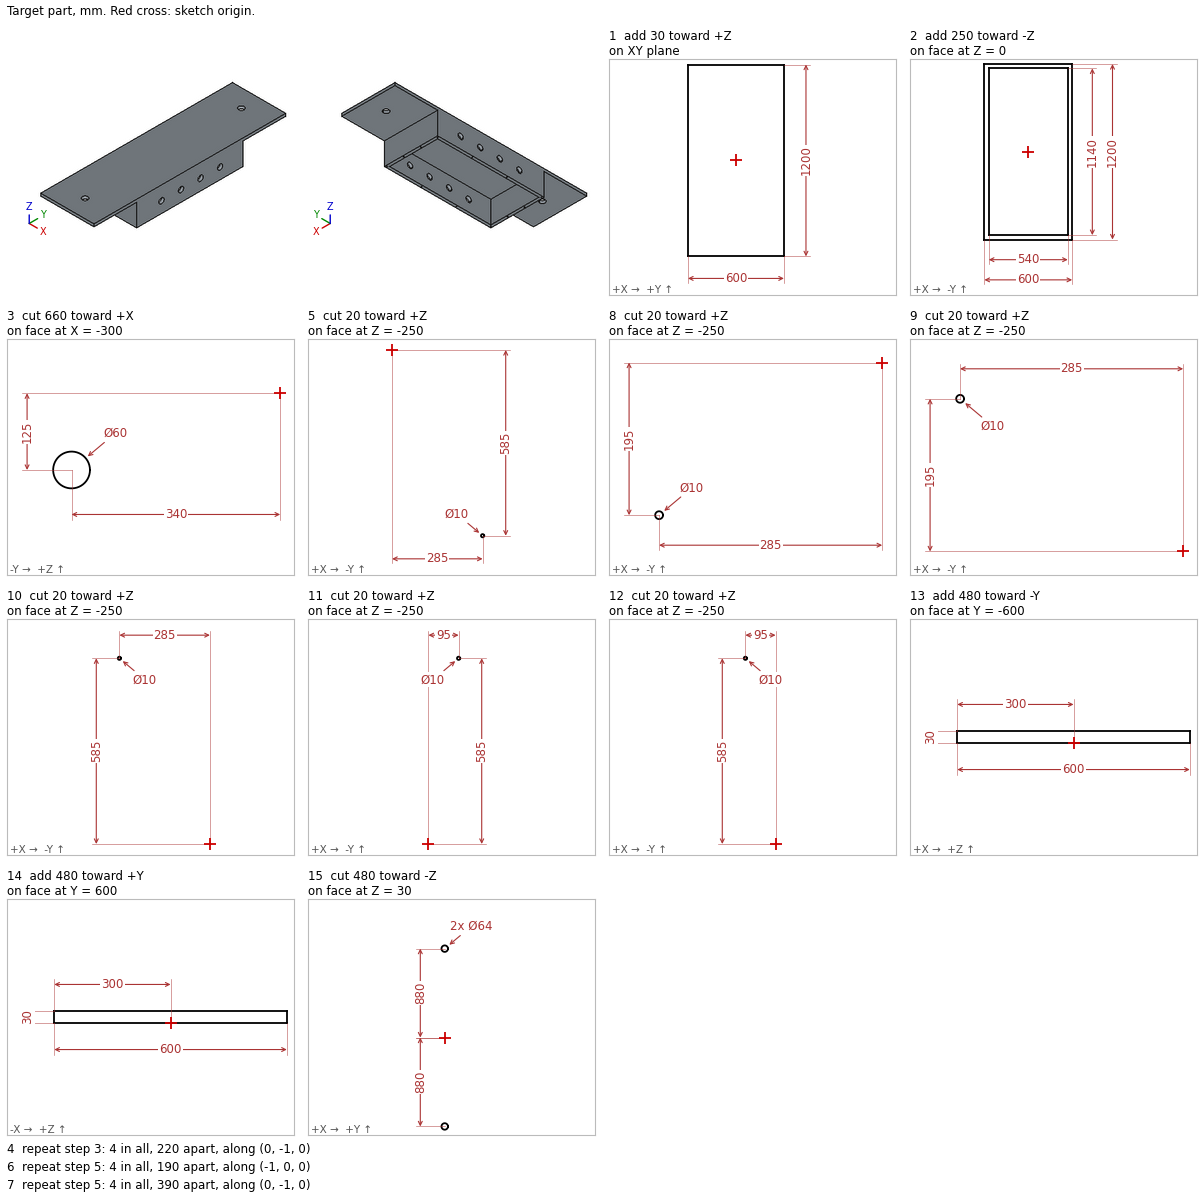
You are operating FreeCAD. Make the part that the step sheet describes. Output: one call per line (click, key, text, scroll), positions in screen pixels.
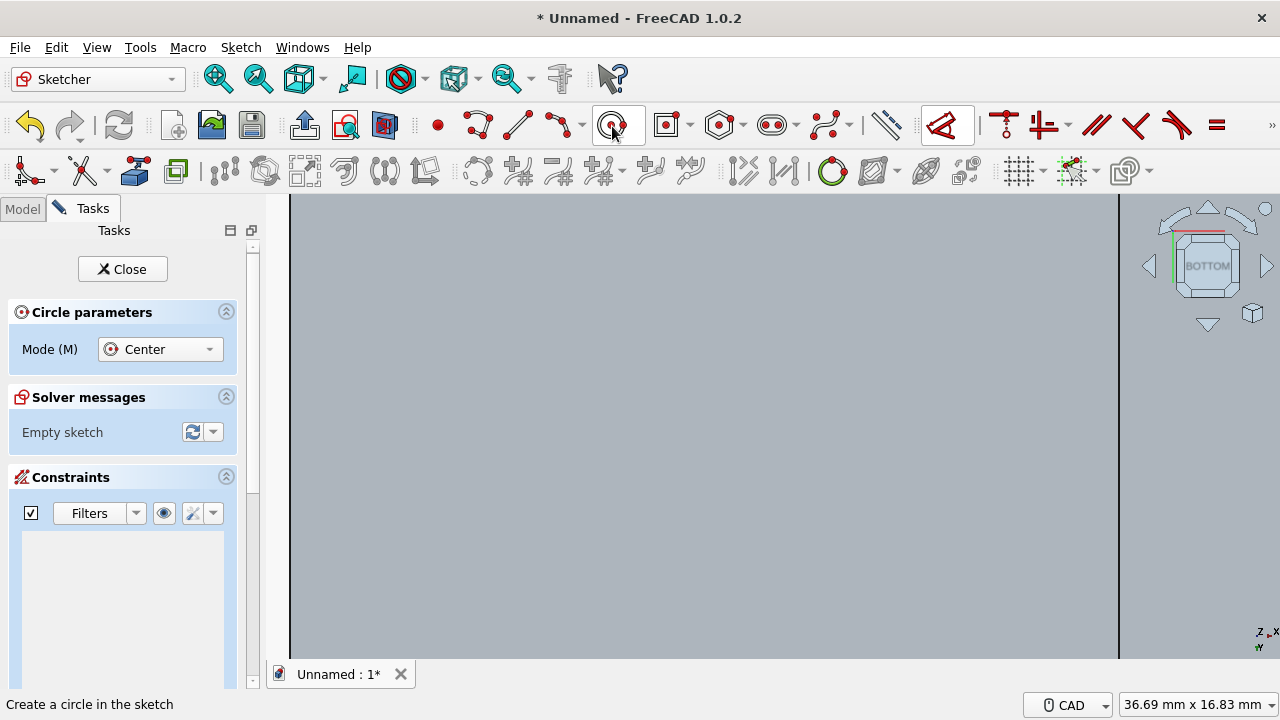
click(704, 426)
move(802, 329)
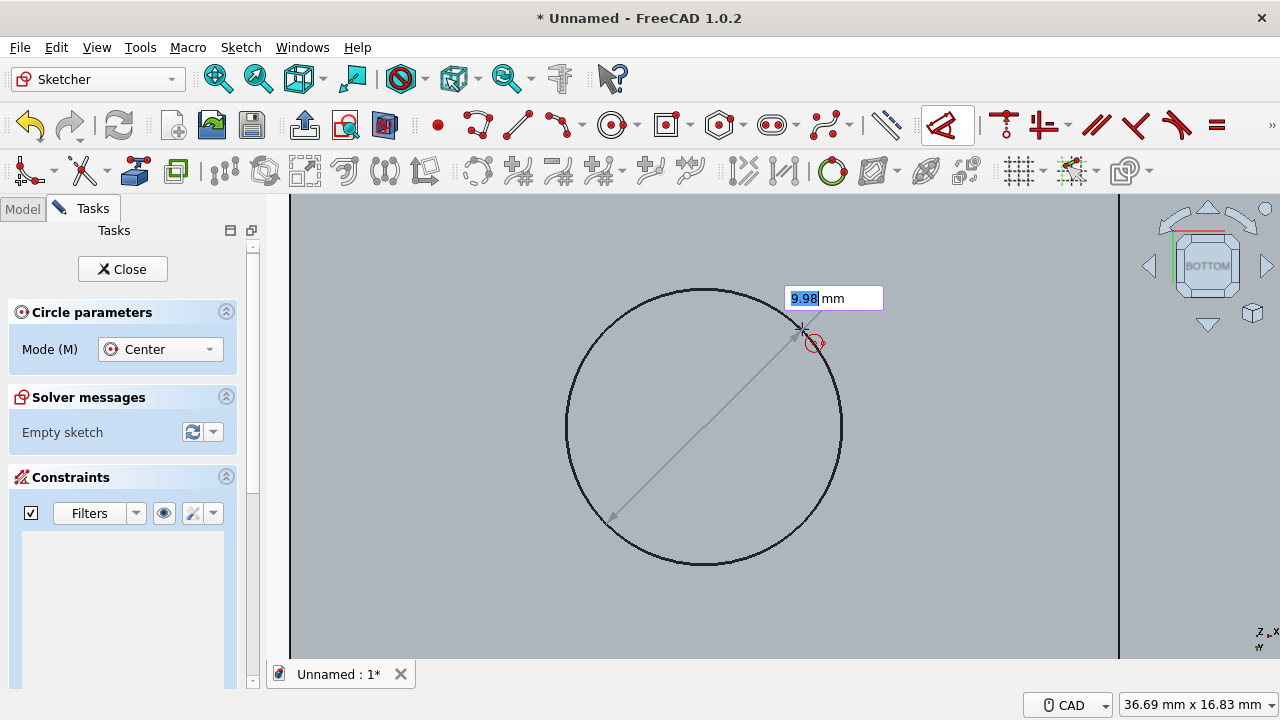
text(10)
key(Return)
key(Escape)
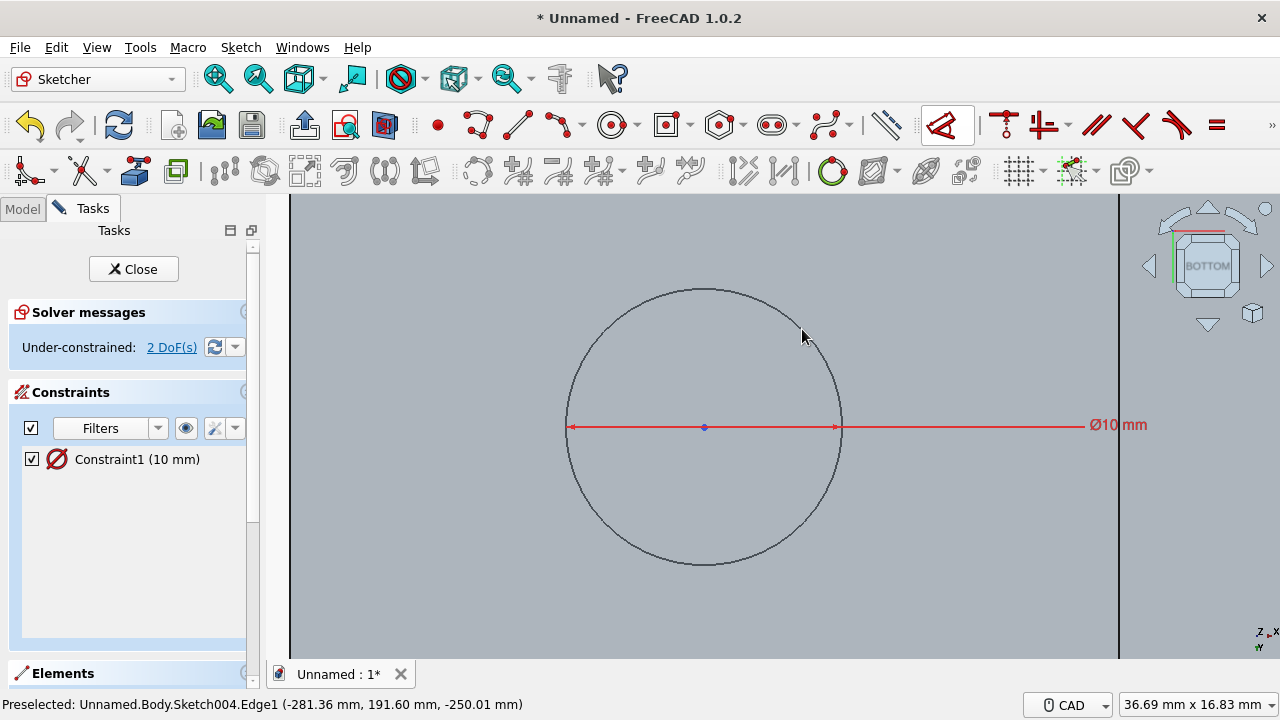
click(704, 427)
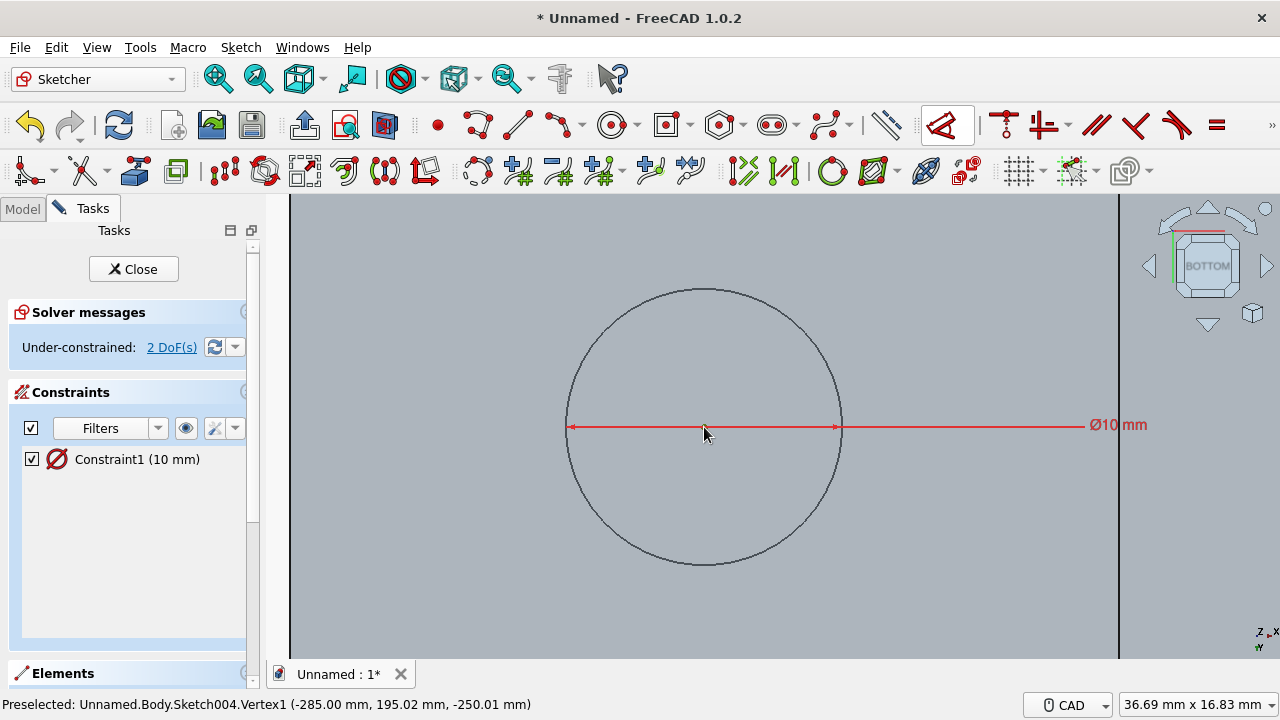
click(968, 126)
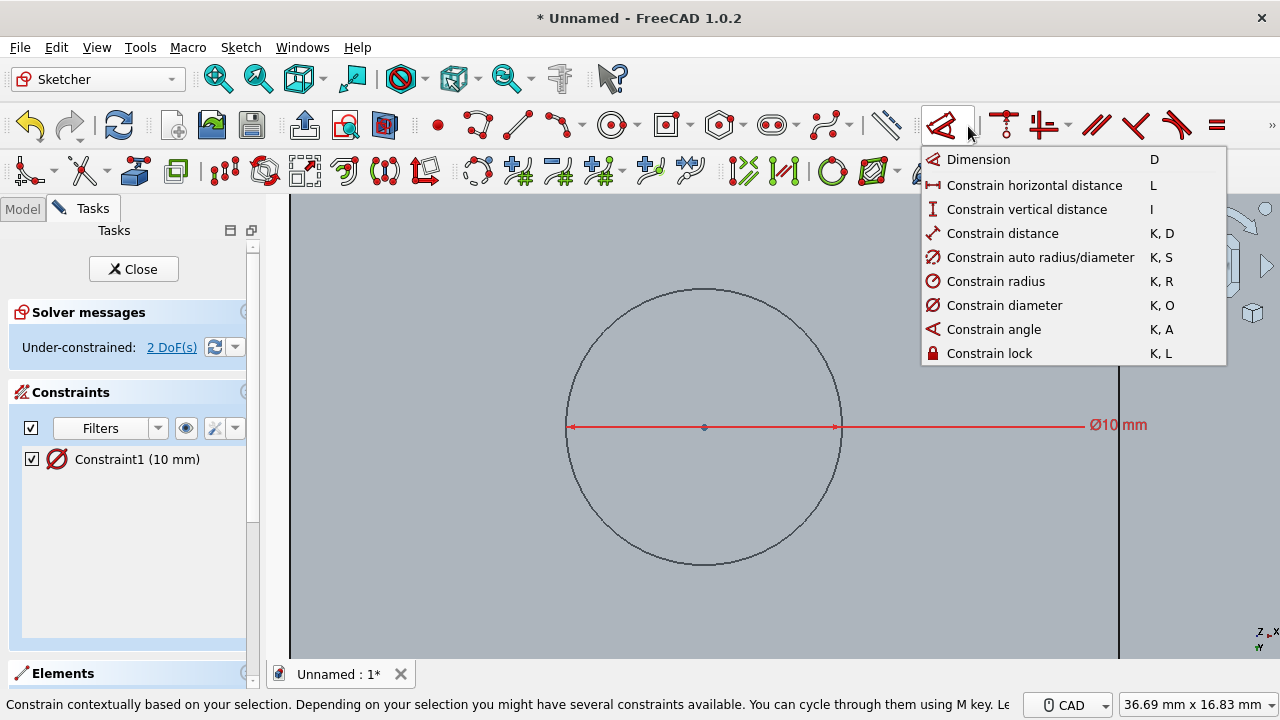
click(1074, 185)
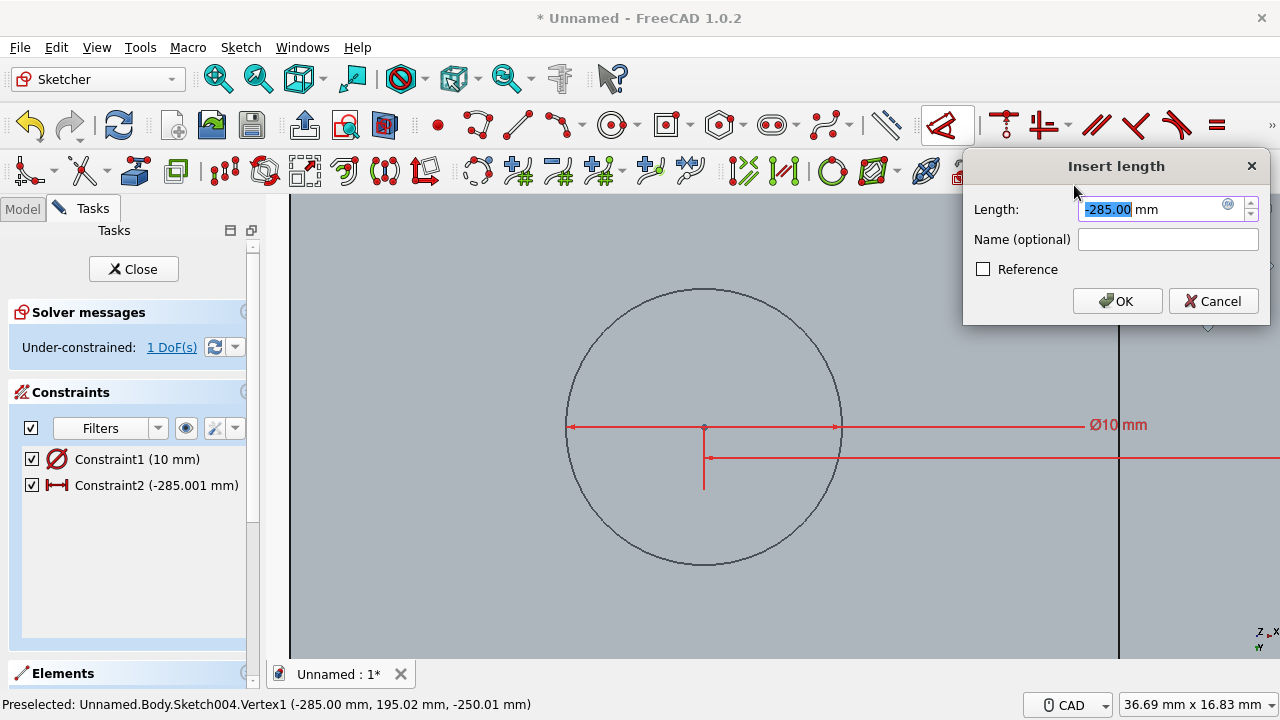
text(-285)
key(Return)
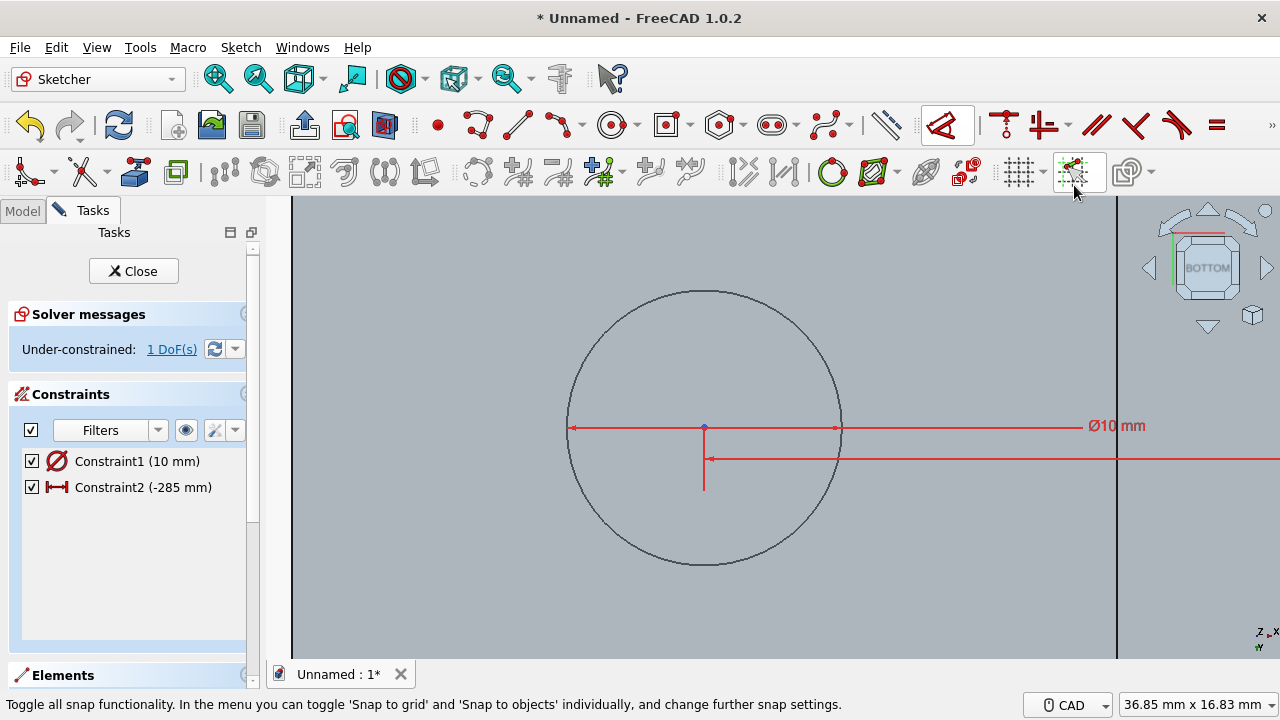
click(704, 428)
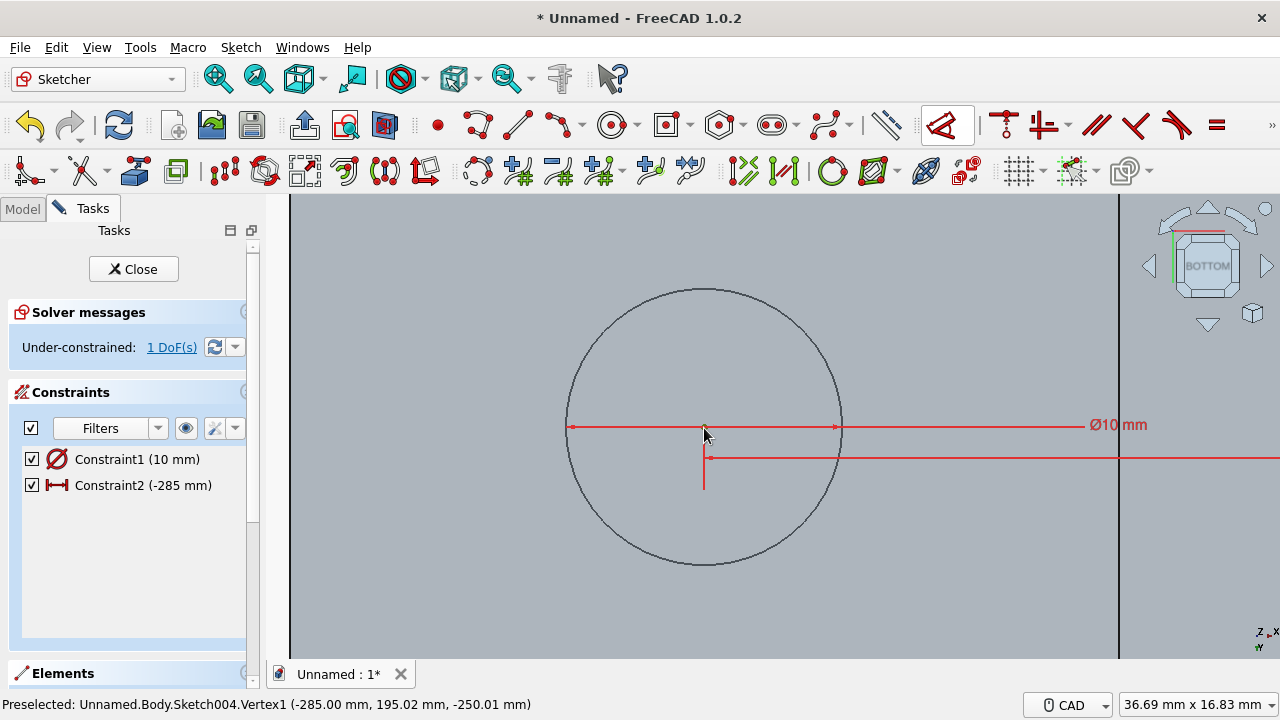
click(968, 126)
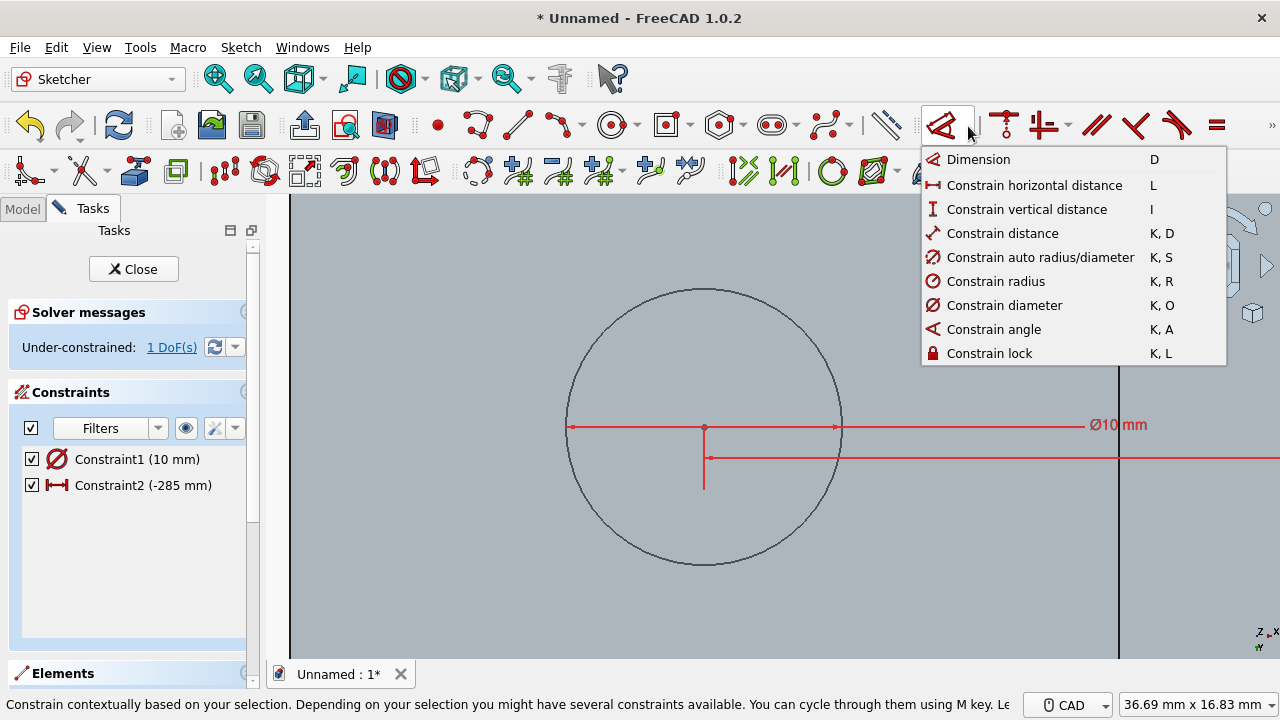
click(1074, 209)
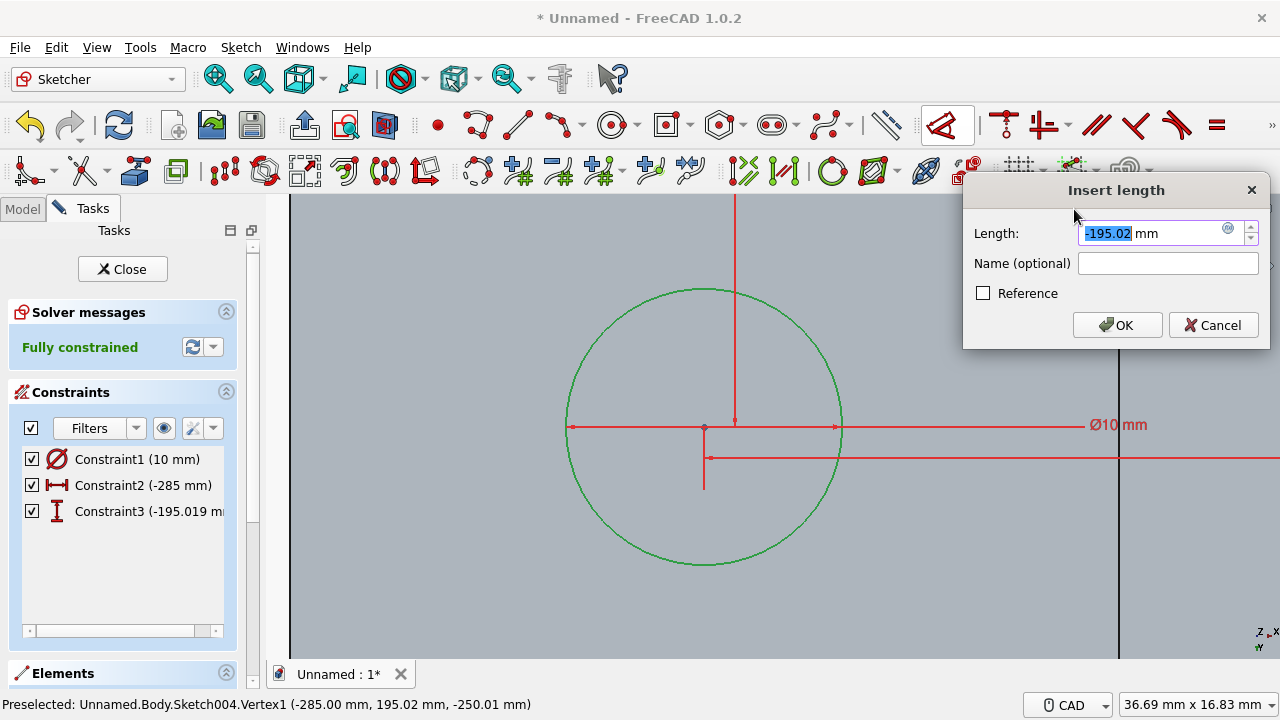
text(-195)
key(Return)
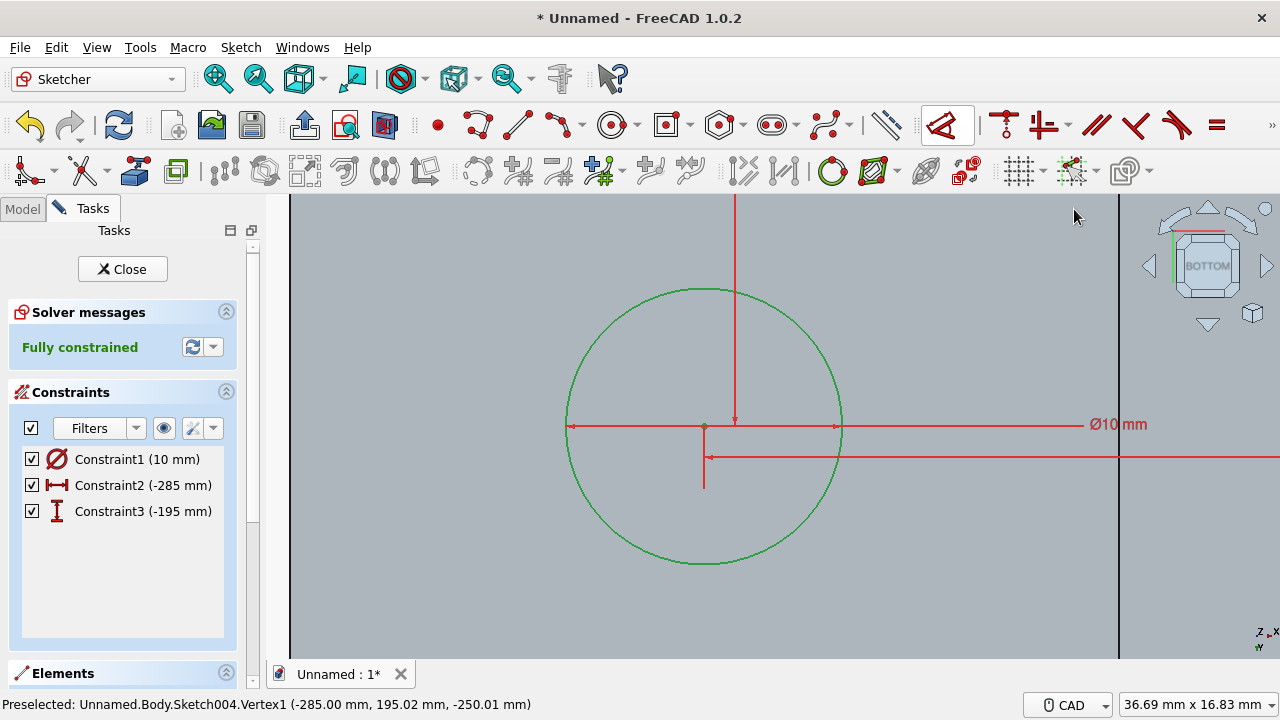
click(123, 269)